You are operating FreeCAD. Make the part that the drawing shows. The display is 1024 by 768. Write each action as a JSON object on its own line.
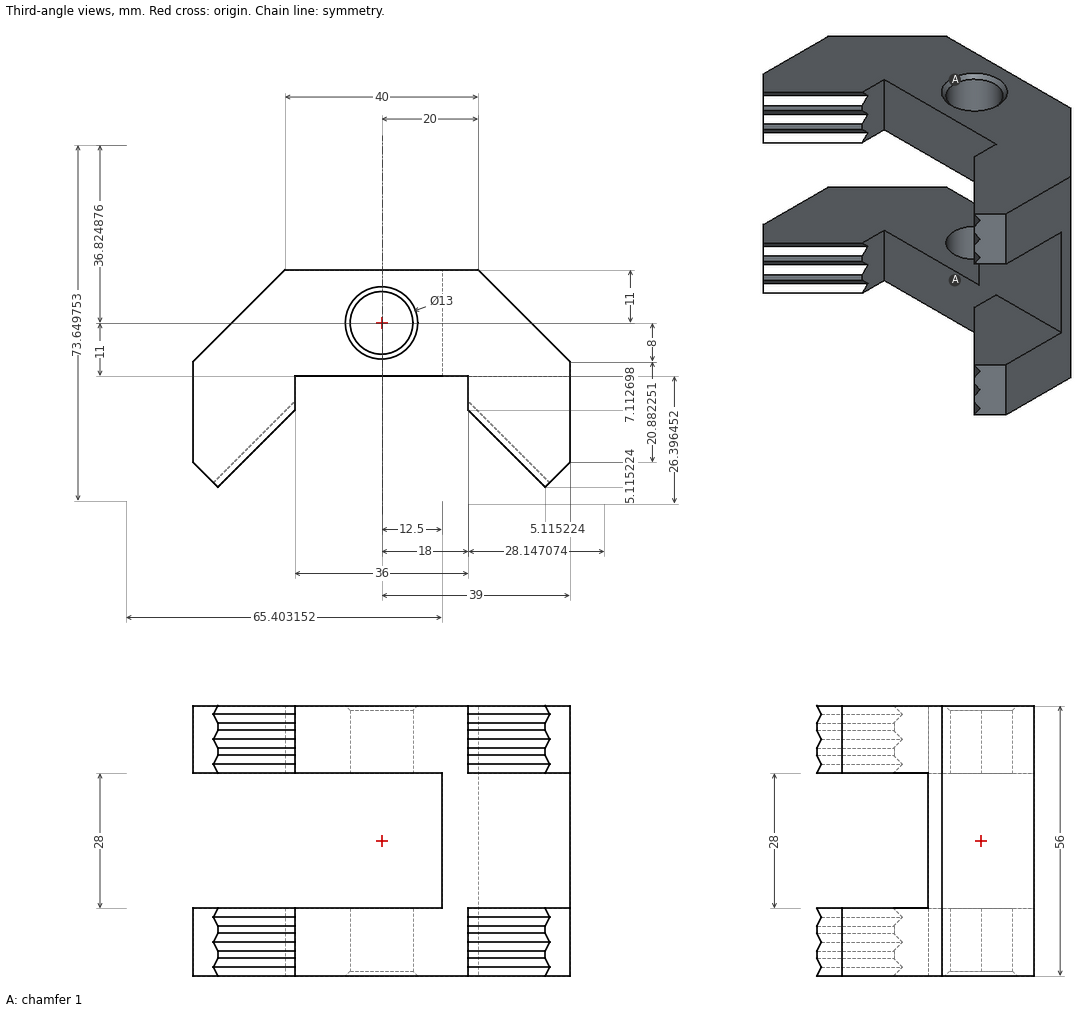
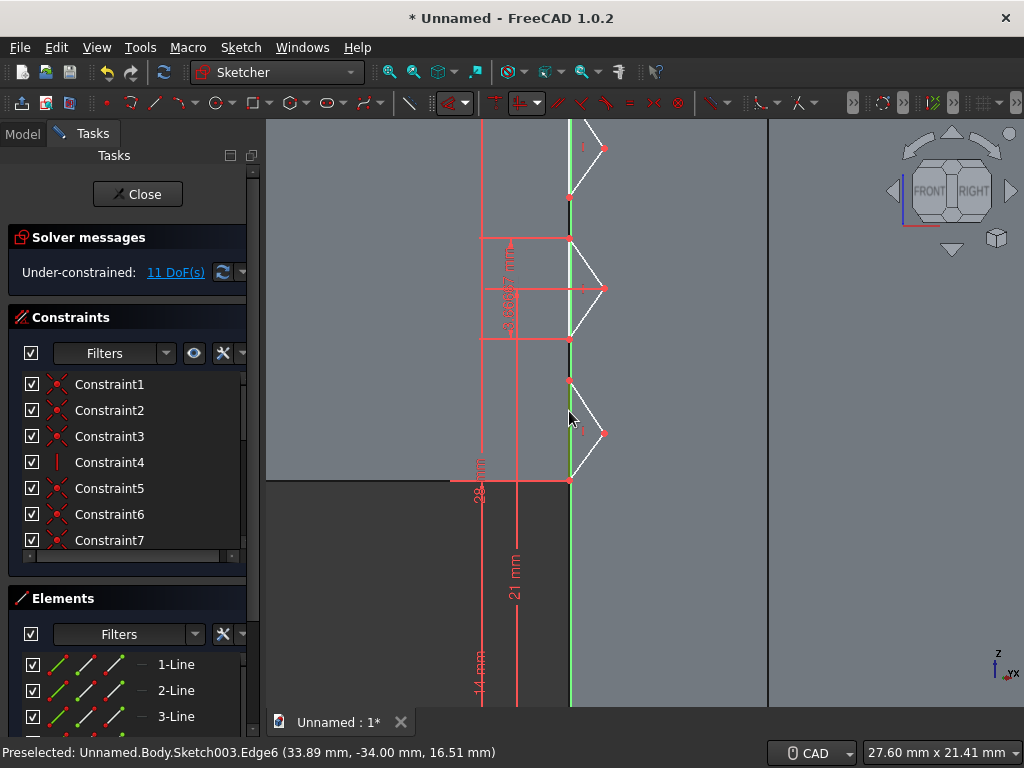
{"action": "key", "text": "i"}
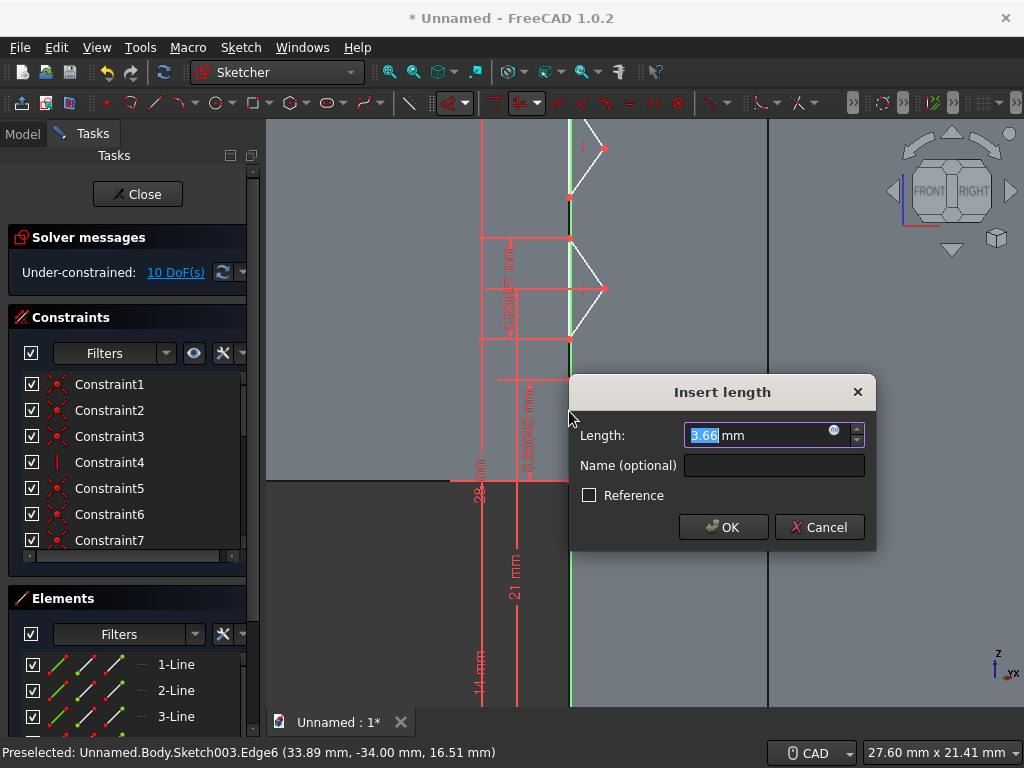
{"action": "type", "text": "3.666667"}
{"action": "key", "text": "Return"}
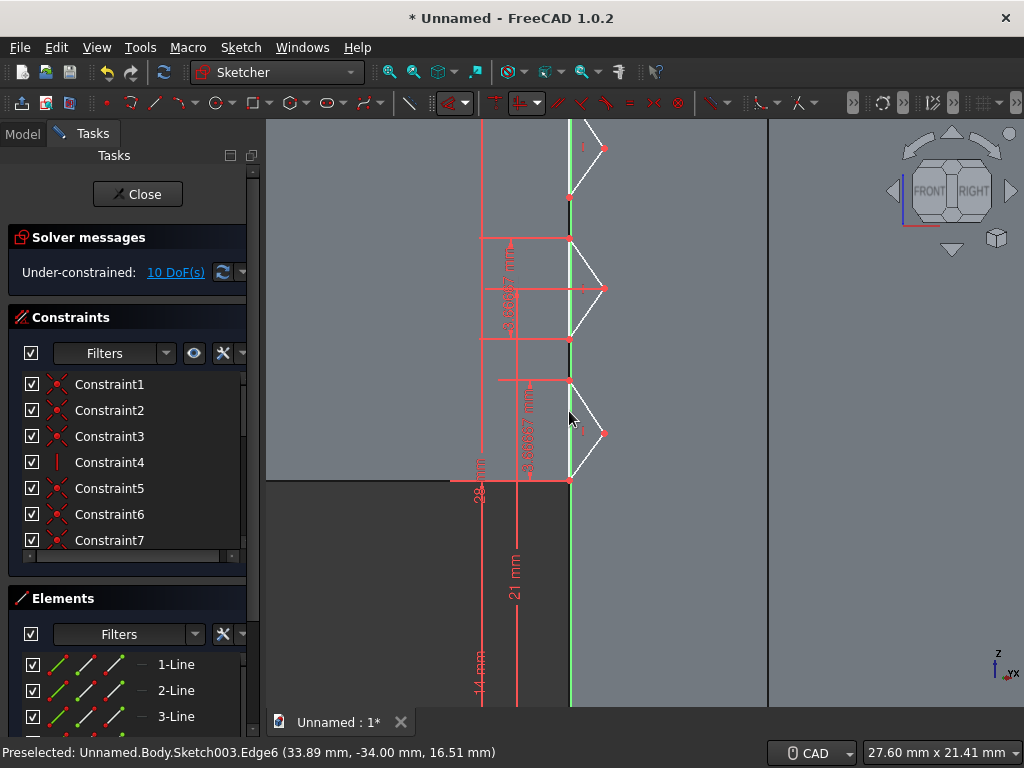
{"action": "left_click", "coordinate": [569, 167]}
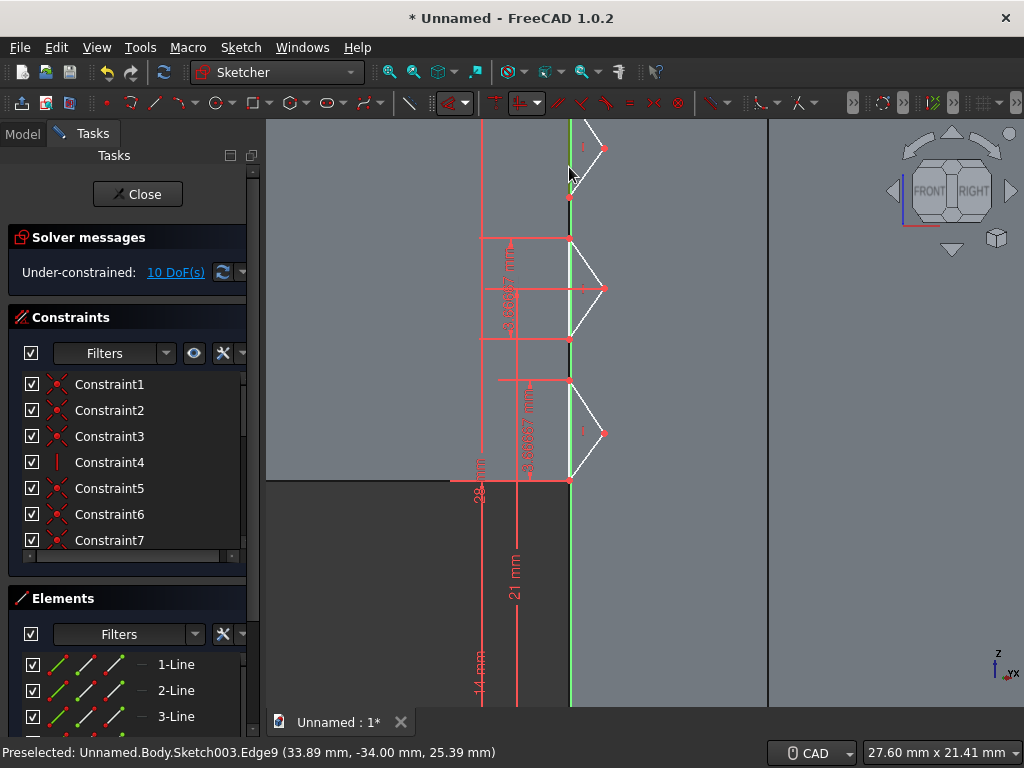
{"action": "left_click", "coordinate": [468, 104]}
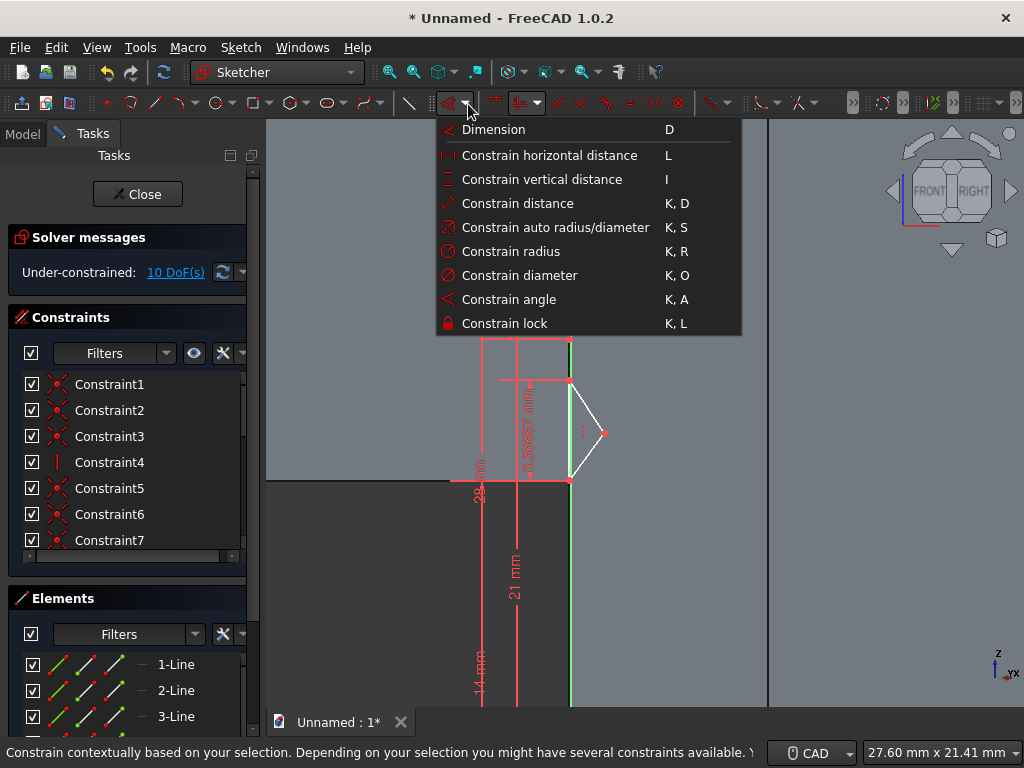
{"action": "left_click", "coordinate": [589, 179]}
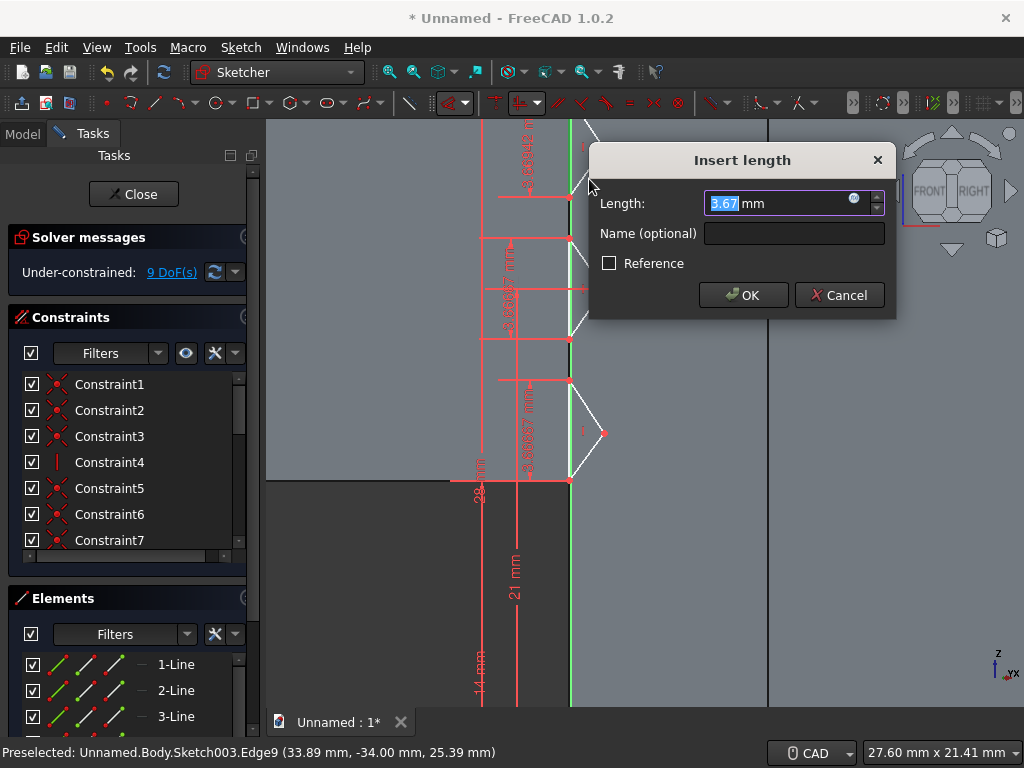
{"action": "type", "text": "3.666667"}
{"action": "key", "text": "Return"}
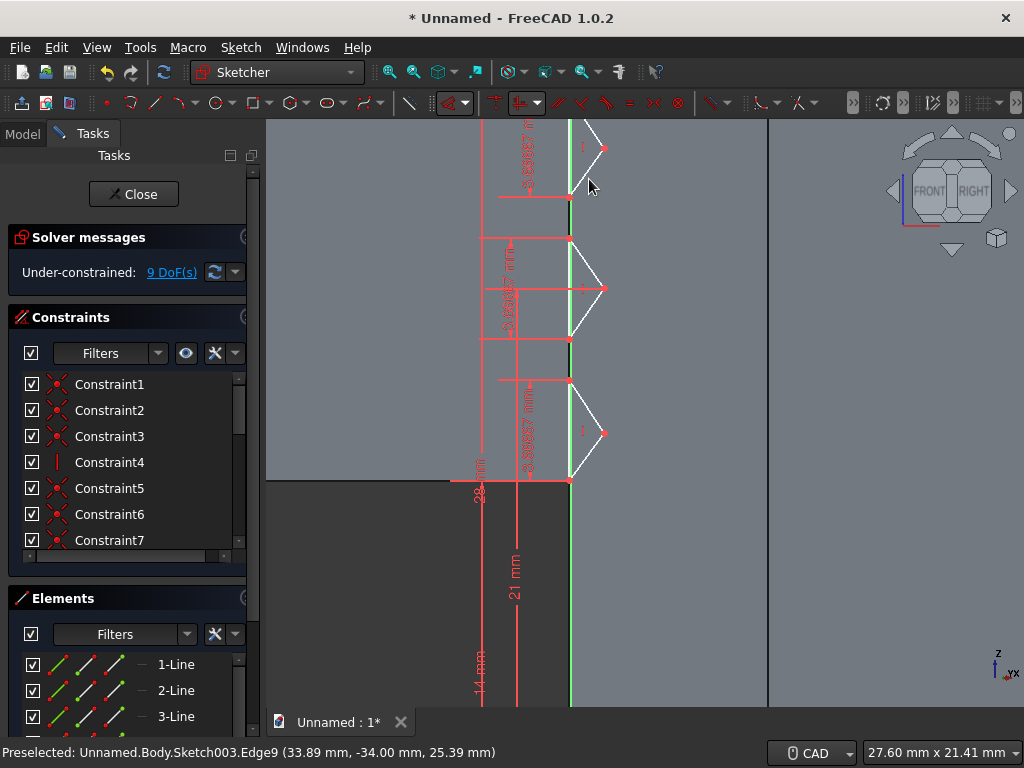
{"action": "scroll", "coordinate": [569, 339], "scroll_direction": "up", "scroll_amount": 15}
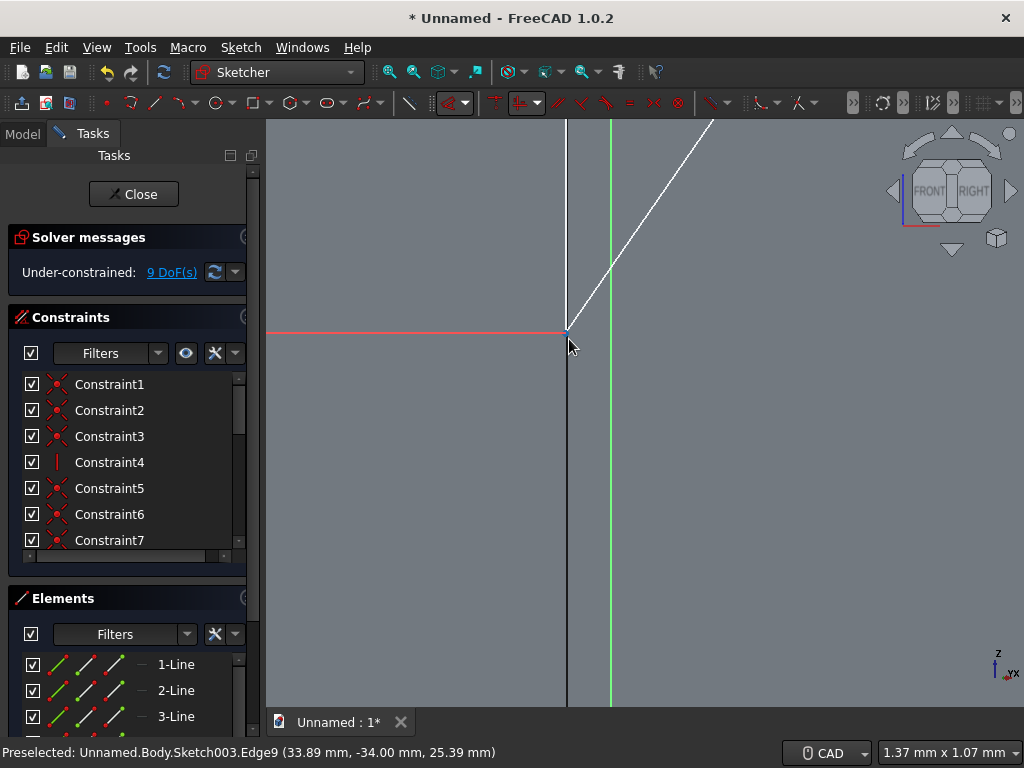
{"action": "left_click", "coordinate": [566, 333]}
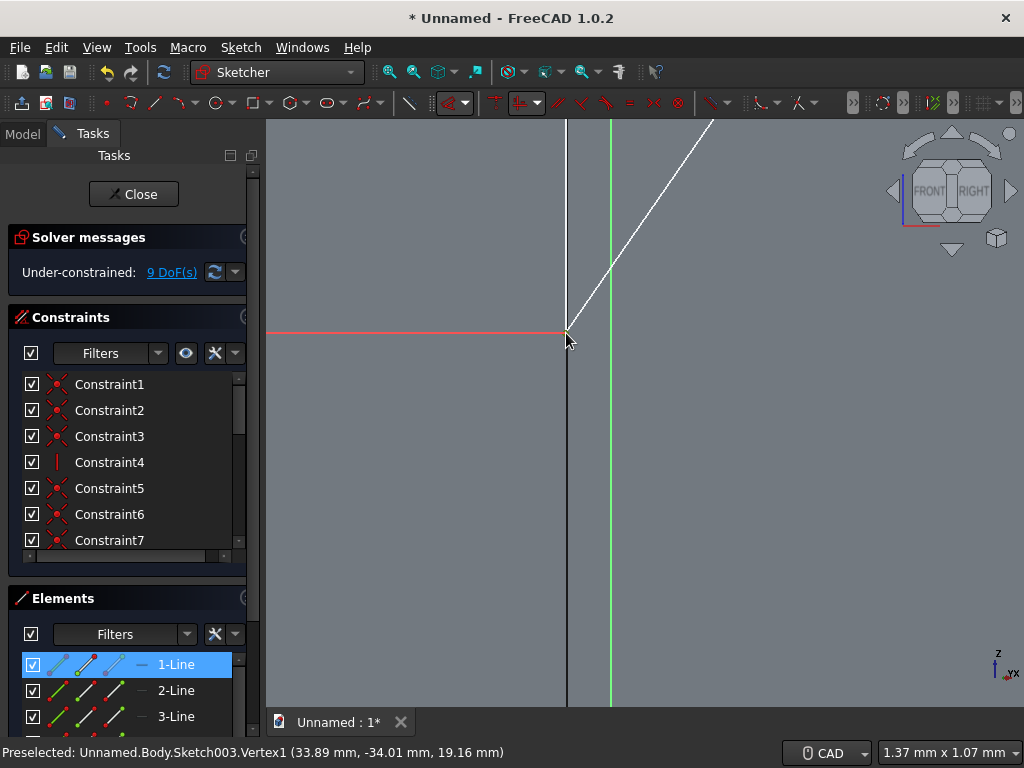
{"action": "left_click", "coordinate": [468, 104]}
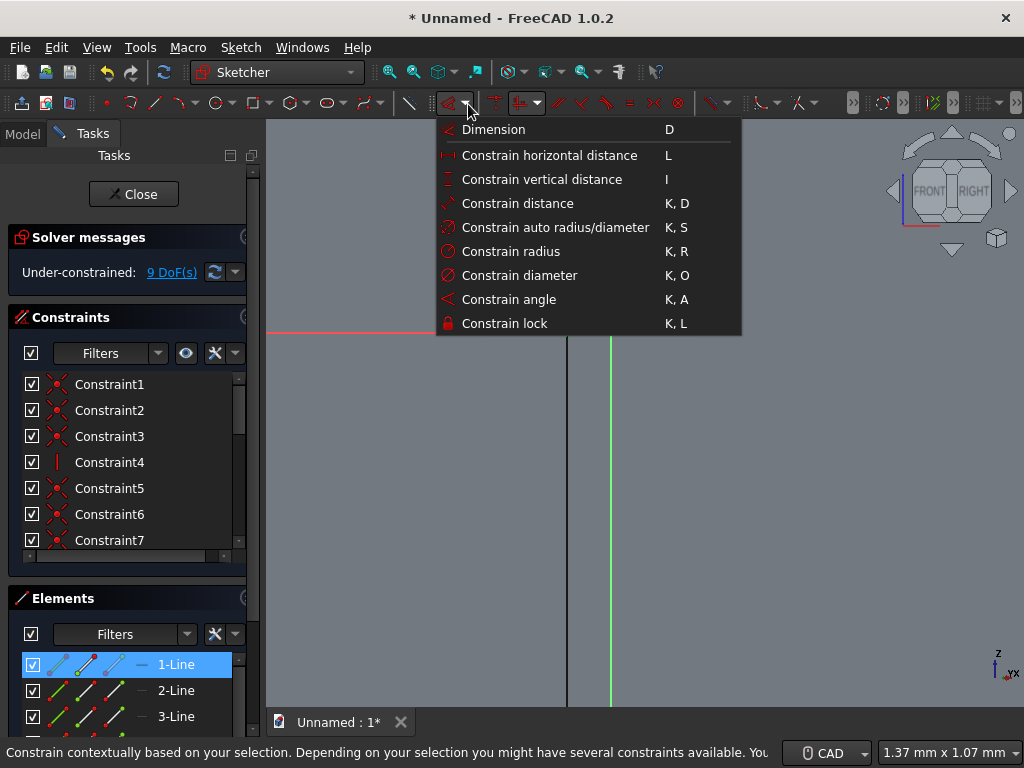
{"action": "left_click", "coordinate": [589, 155]}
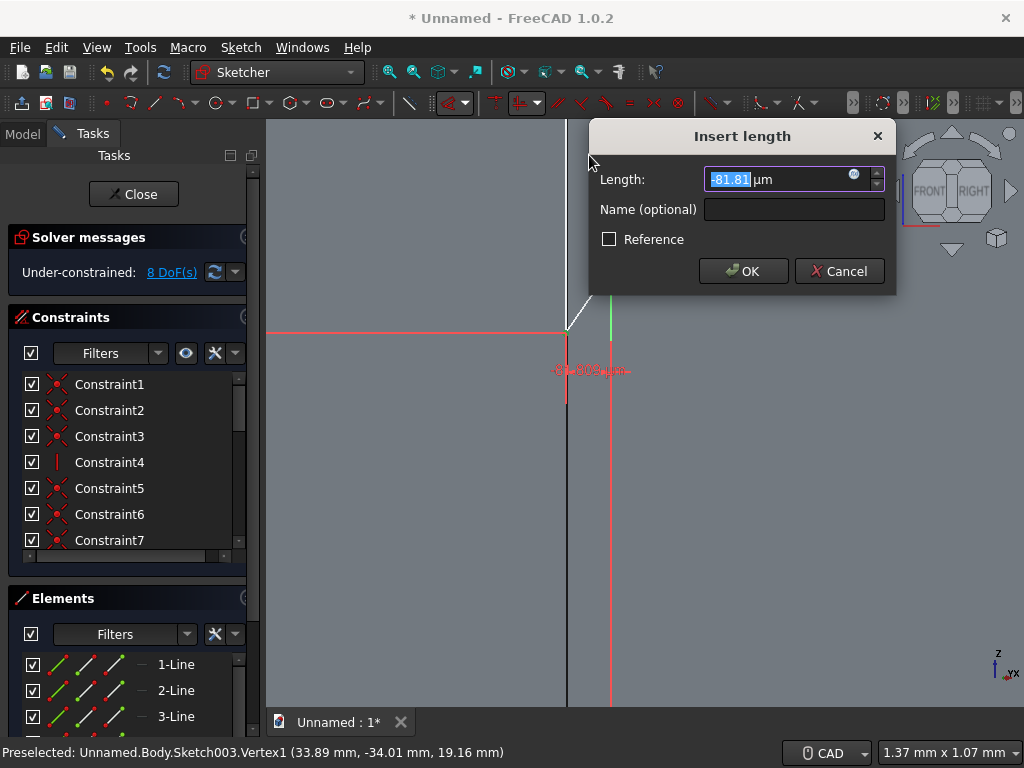
{"action": "key", "text": "ctrl+a"}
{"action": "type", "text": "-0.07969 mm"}
{"action": "key", "text": "Return"}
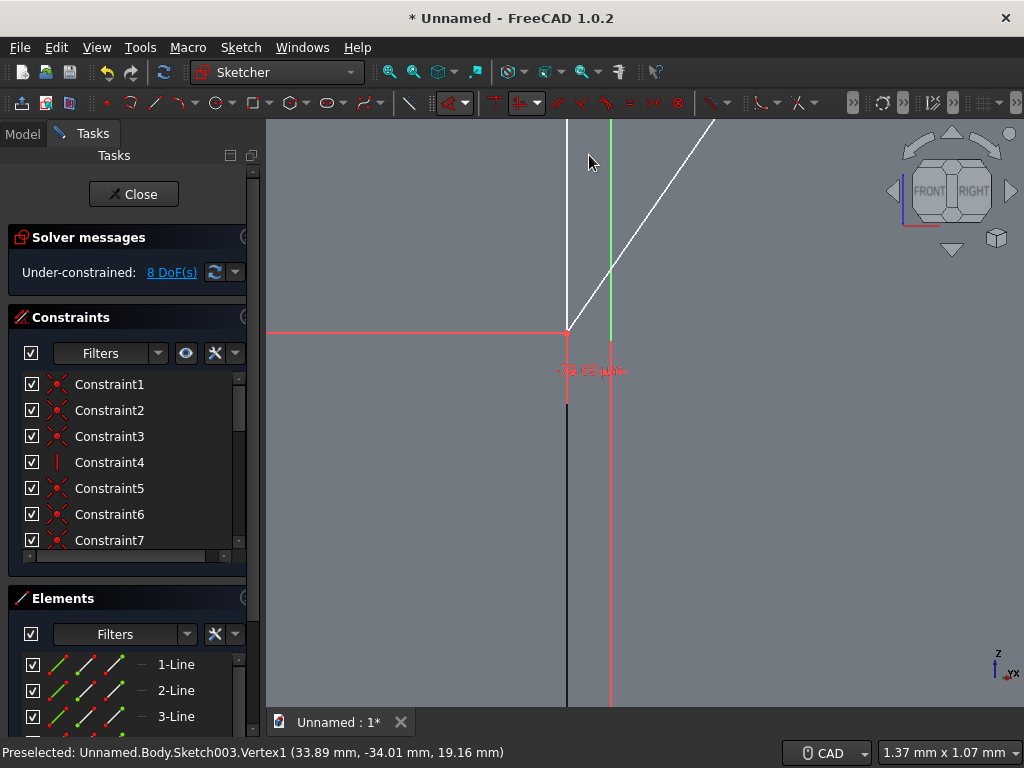
{"action": "scroll", "coordinate": [567, 335], "scroll_direction": "down", "scroll_amount": 18}